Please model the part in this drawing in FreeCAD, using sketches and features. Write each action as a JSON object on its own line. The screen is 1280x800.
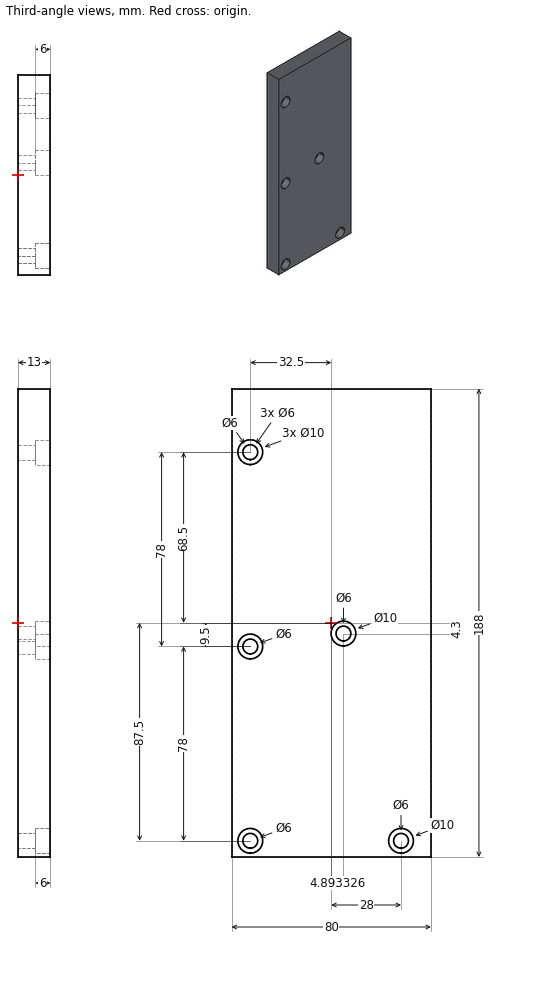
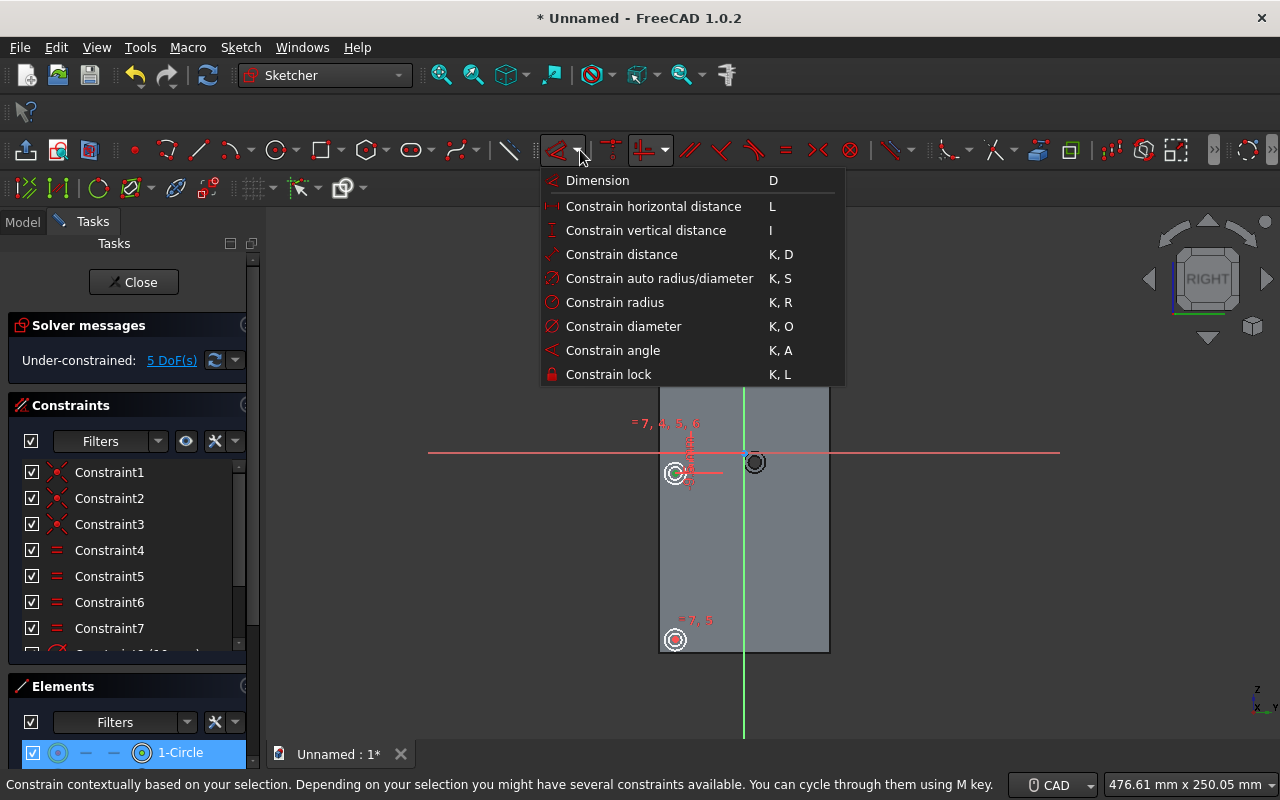
{"action": "left_click", "coordinate": [693, 230]}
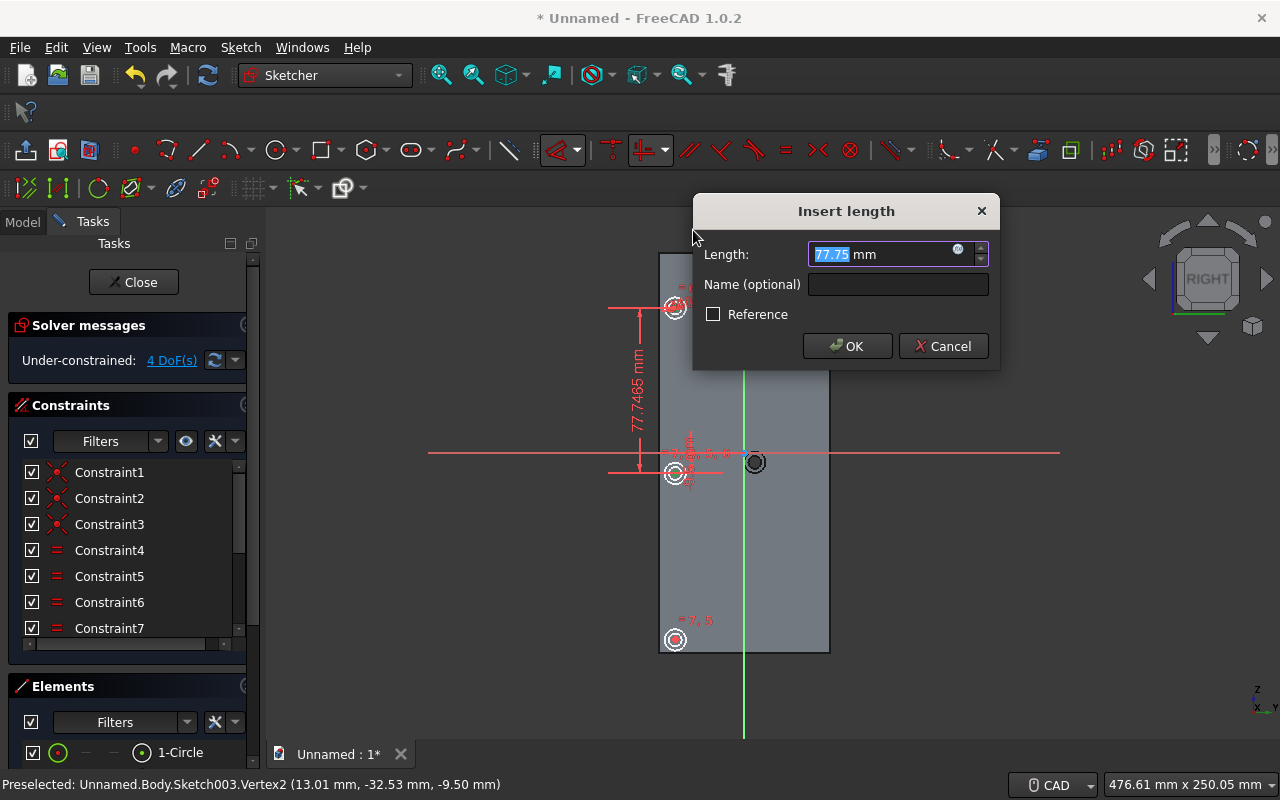
{"action": "type", "text": "78"}
{"action": "key", "text": "Return"}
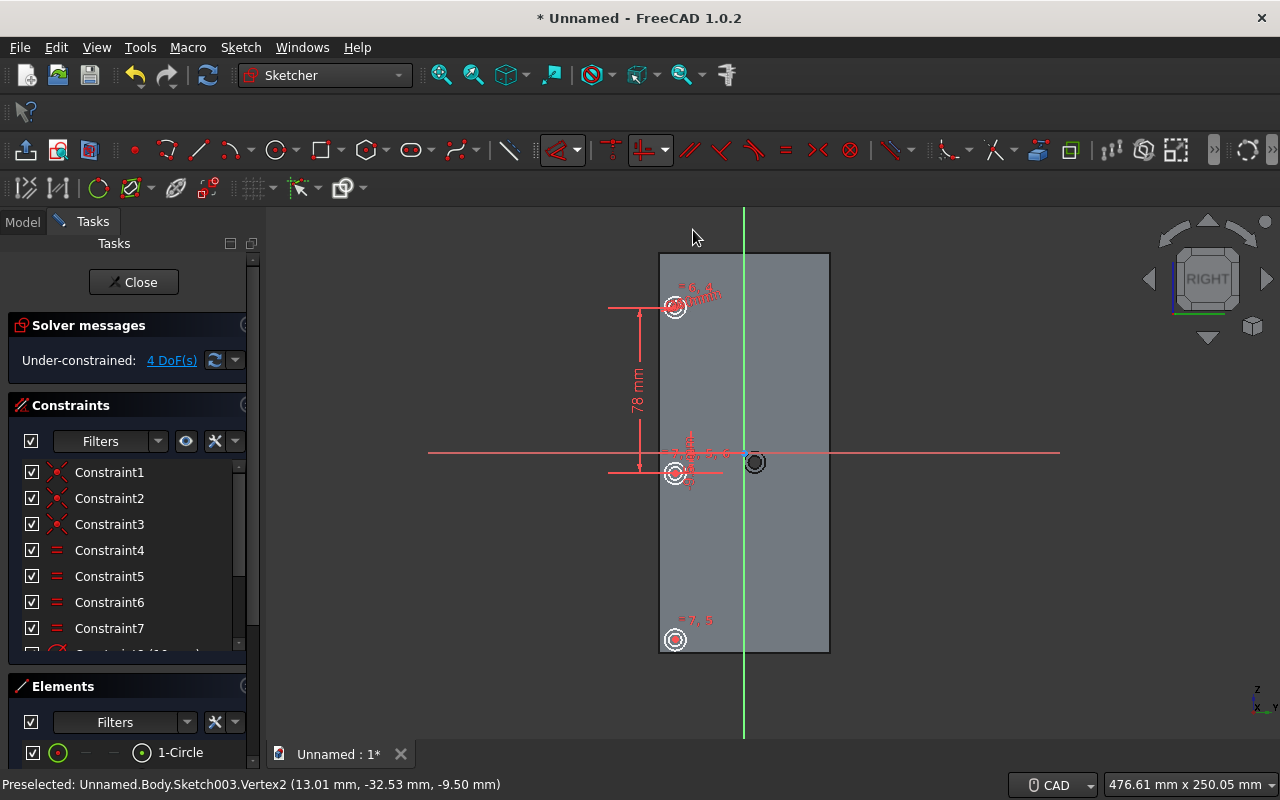
{"action": "left_click", "coordinate": [675, 473]}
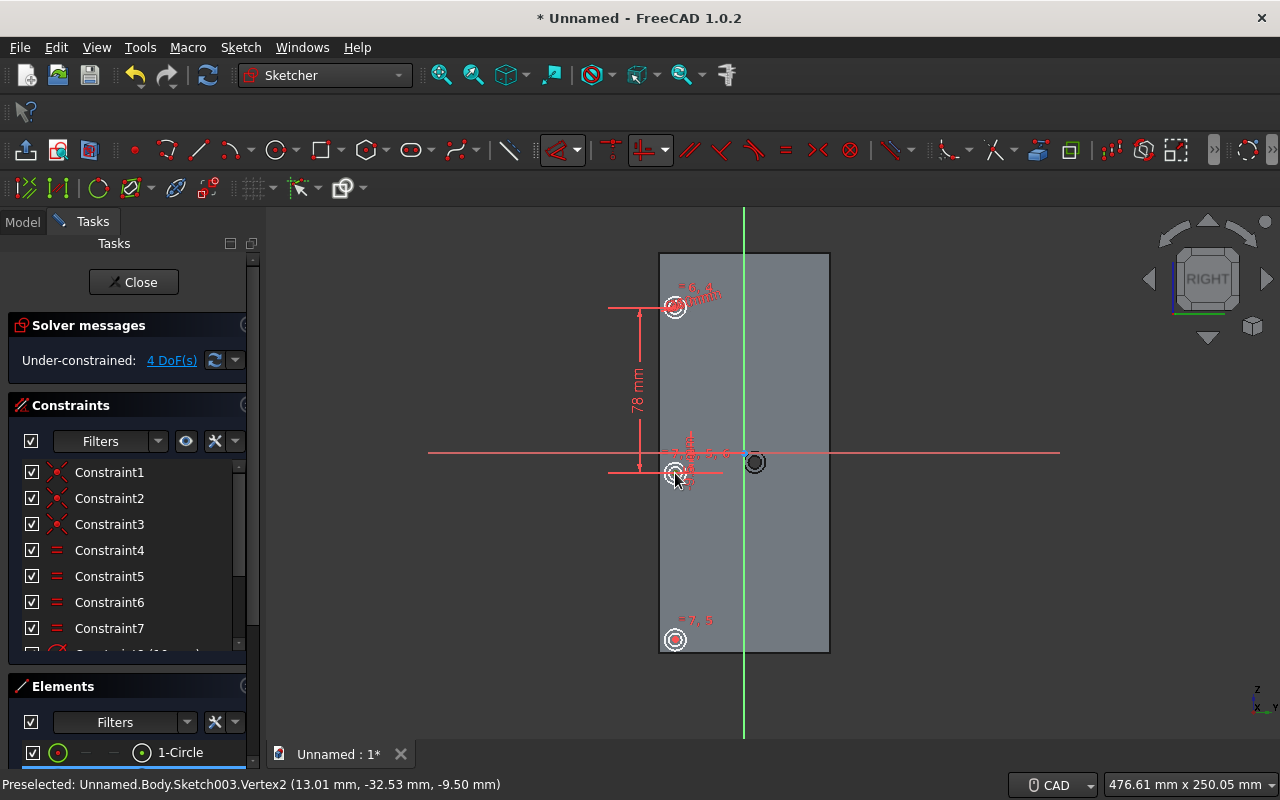
{"action": "left_click", "coordinate": [675, 640]}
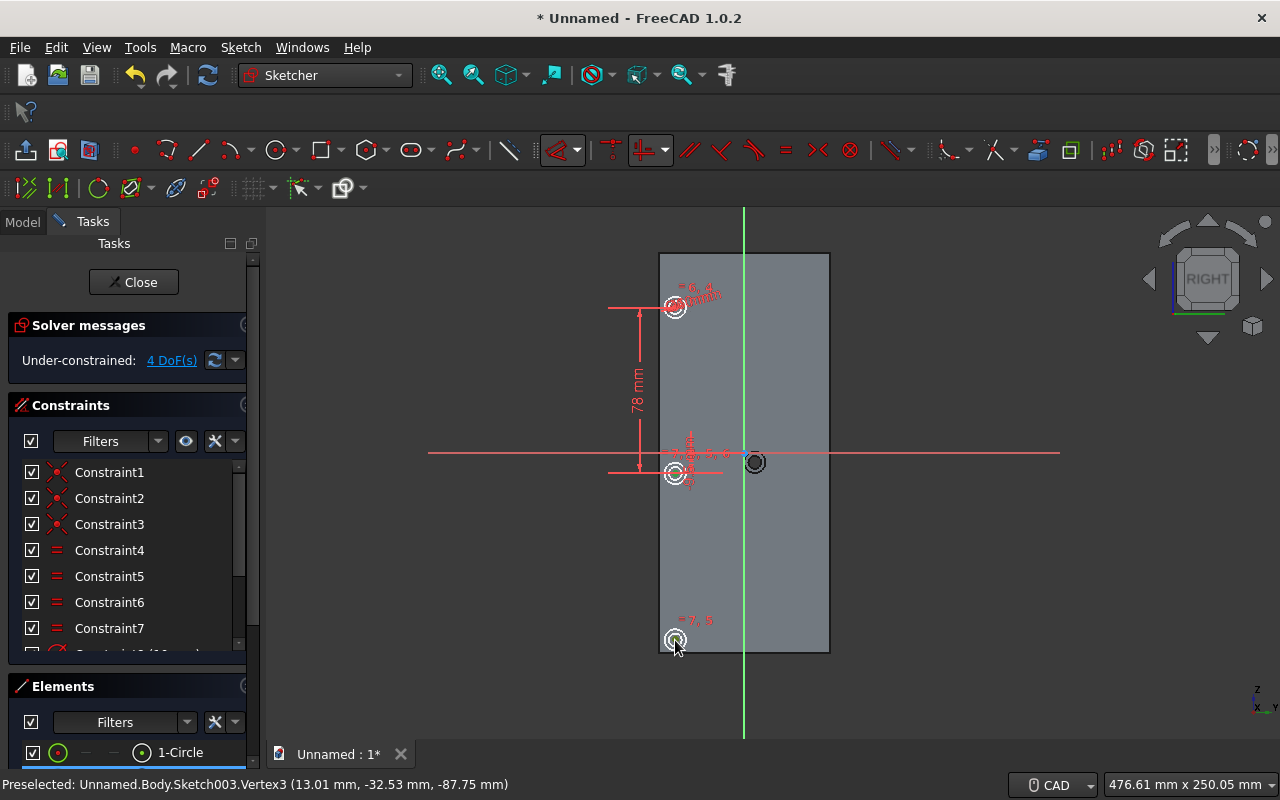
{"action": "key", "text": "i"}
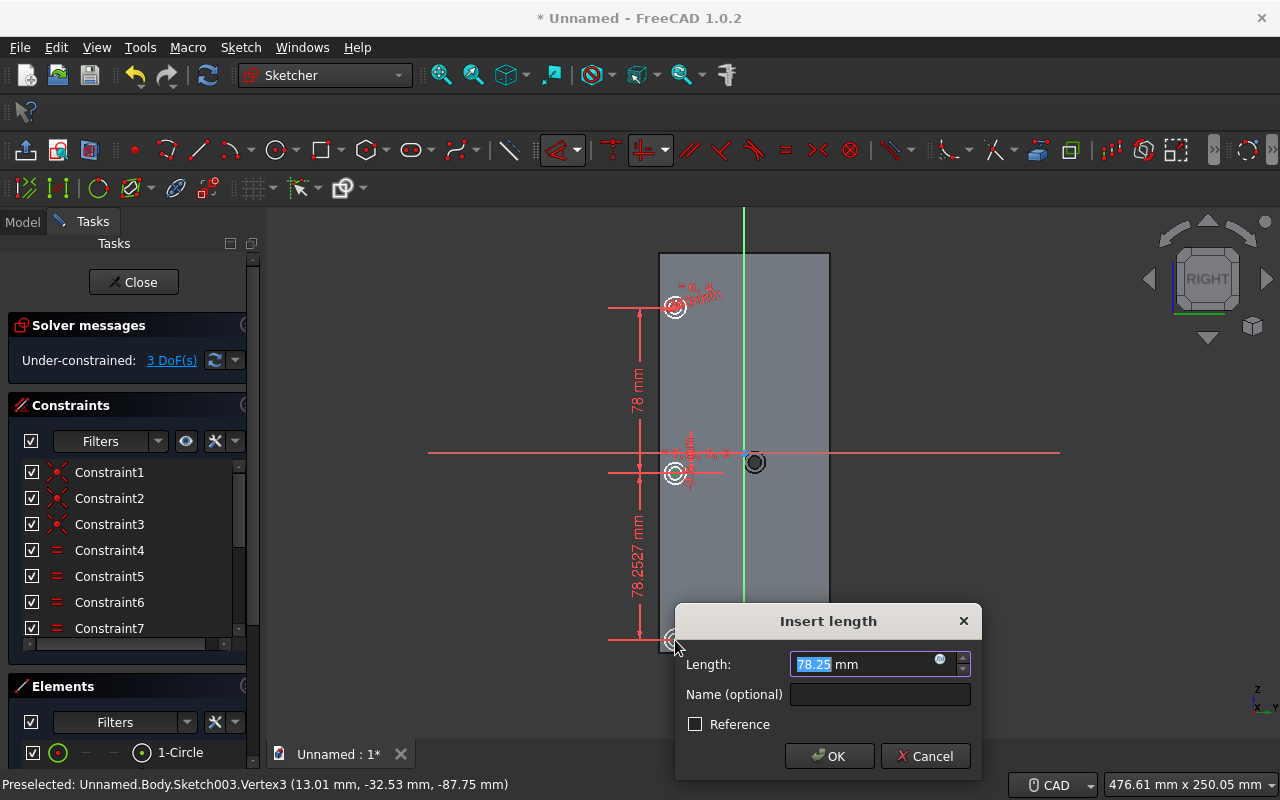
{"action": "type", "text": "78"}
{"action": "key", "text": "Return"}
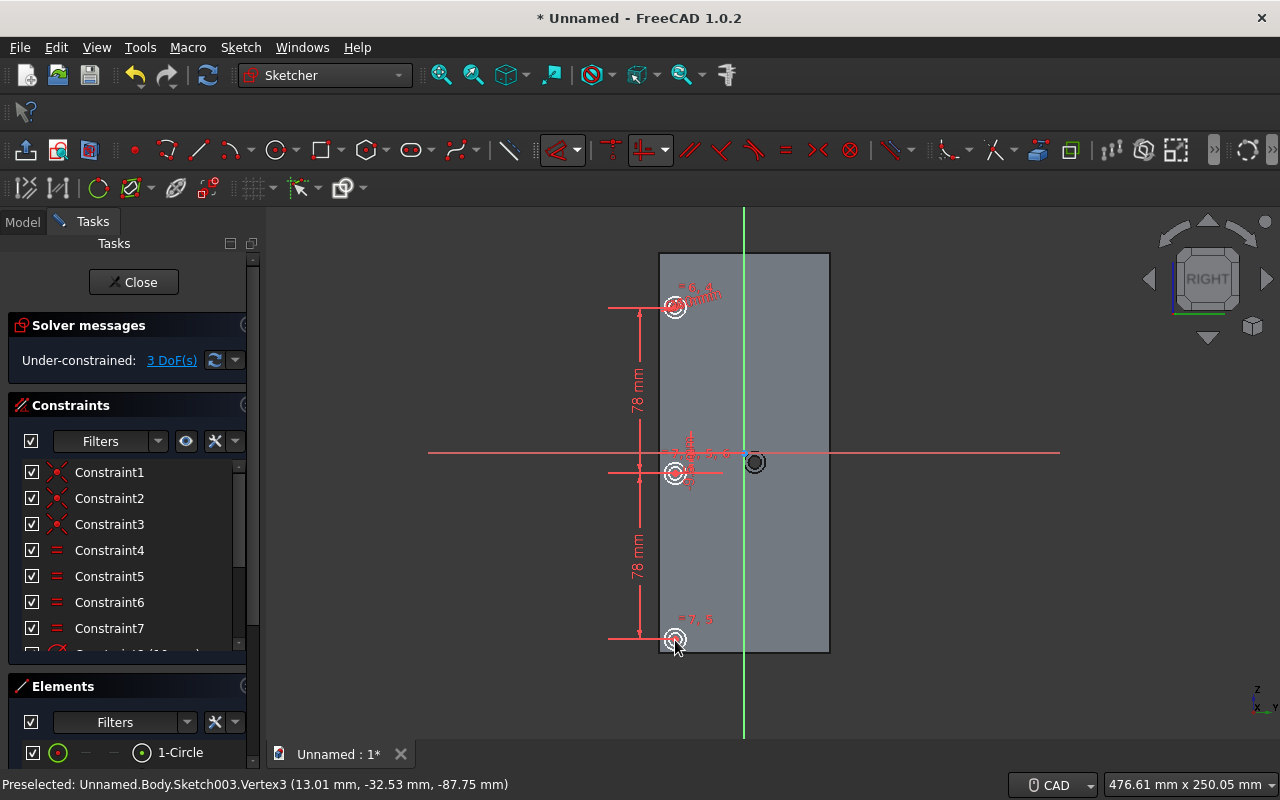
{"action": "left_click", "coordinate": [675, 308]}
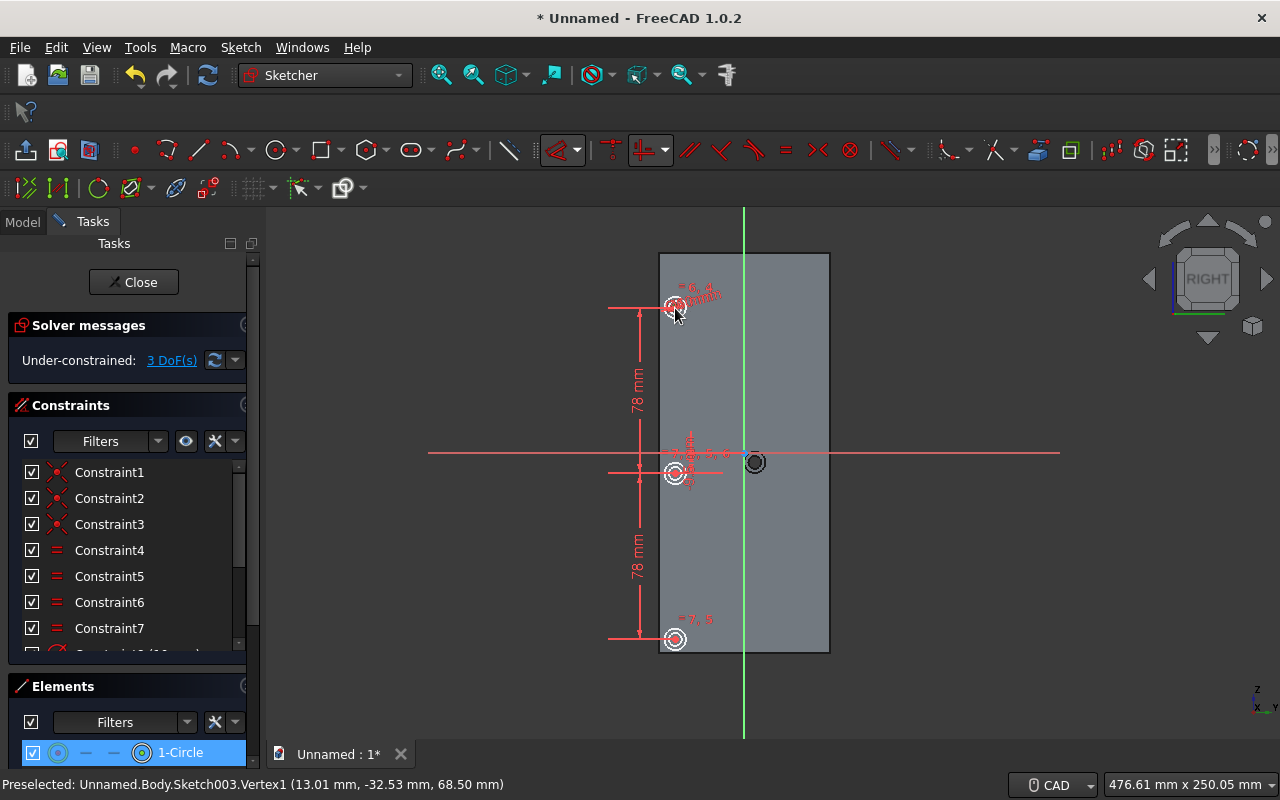
{"action": "key", "text": "l"}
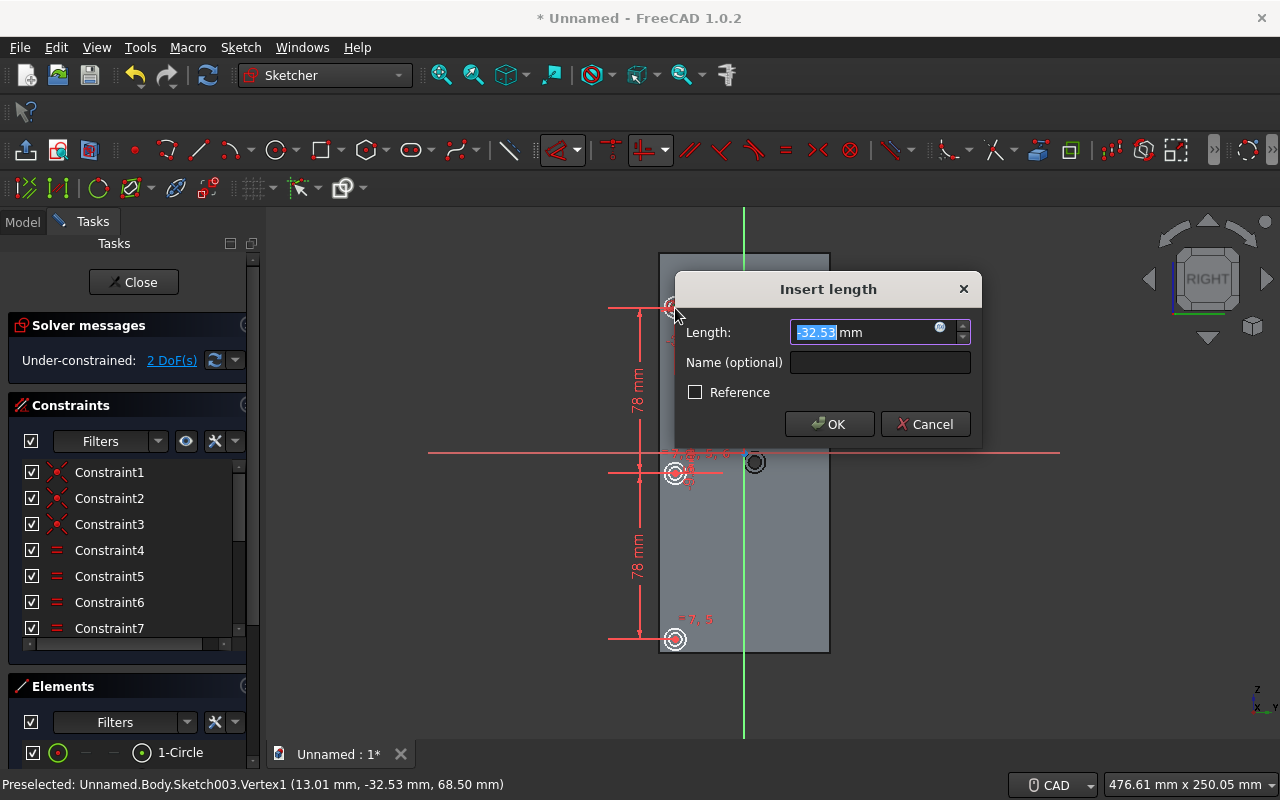
{"action": "type", "text": "-32.5"}
{"action": "key", "text": "Return"}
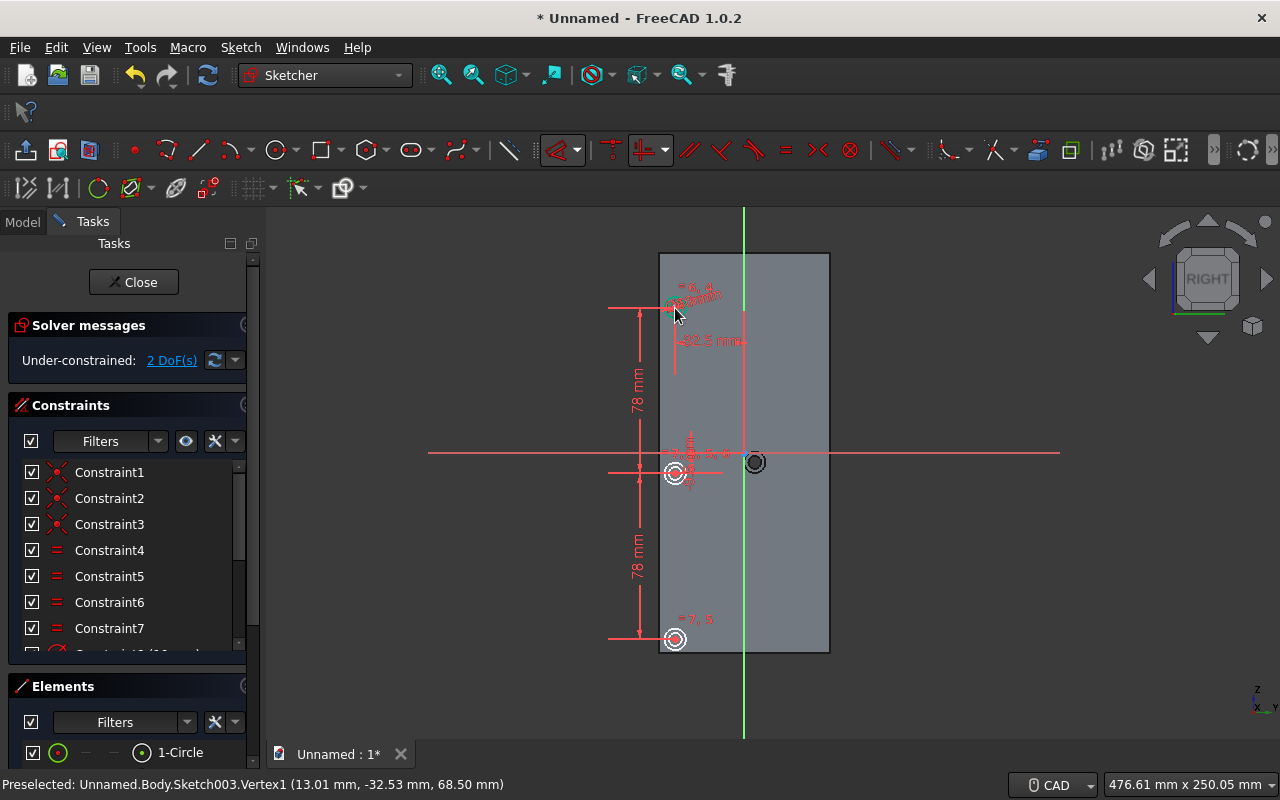
{"action": "left_click", "coordinate": [675, 473]}